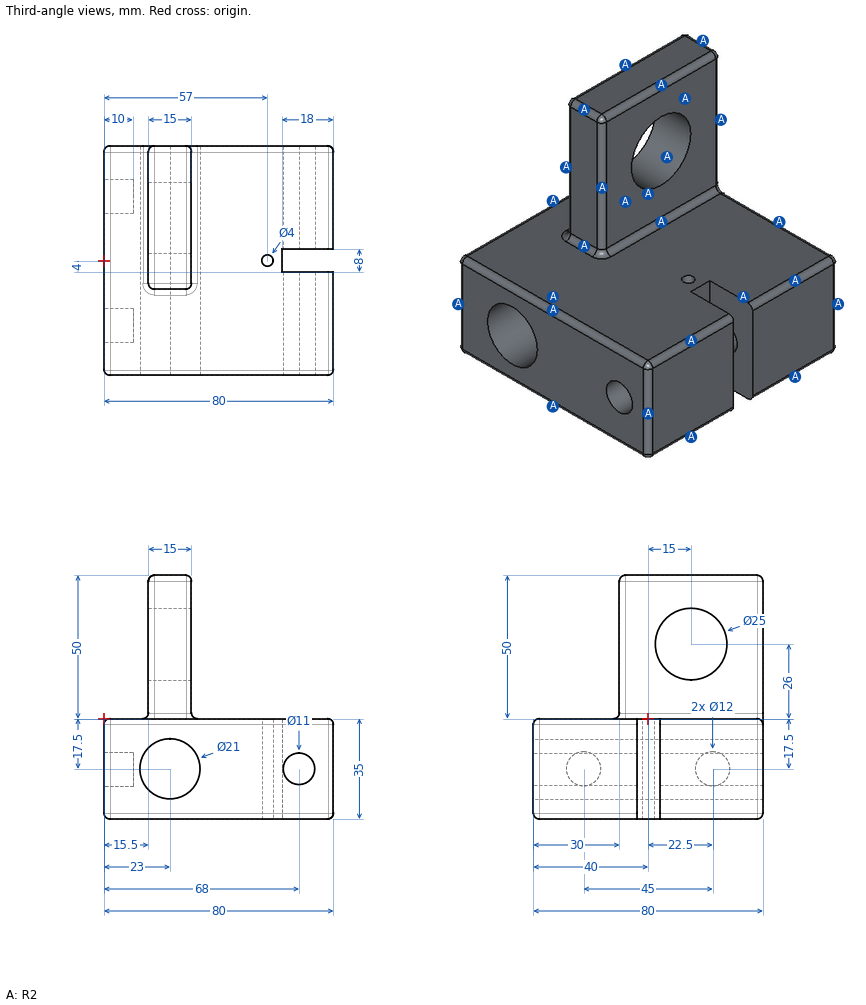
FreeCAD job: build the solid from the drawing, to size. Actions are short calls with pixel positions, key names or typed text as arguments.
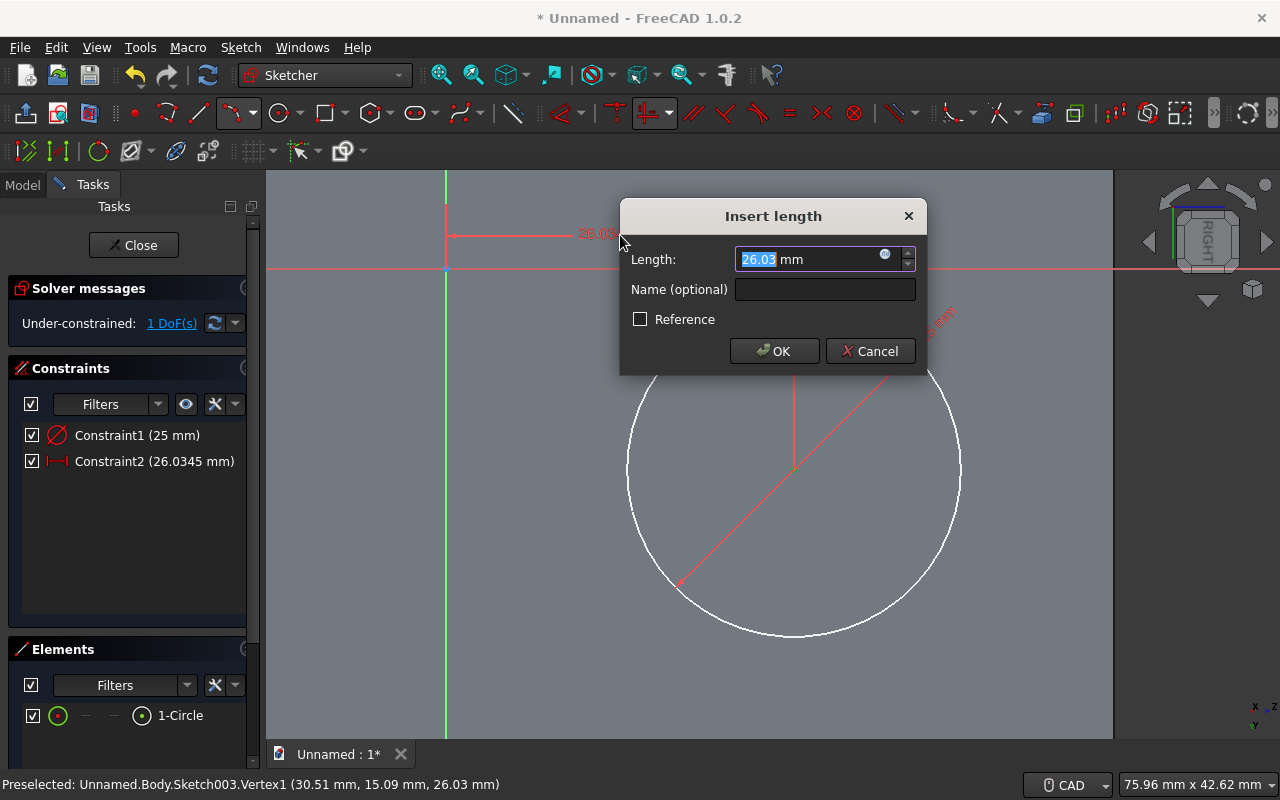
text(26)
key(Return)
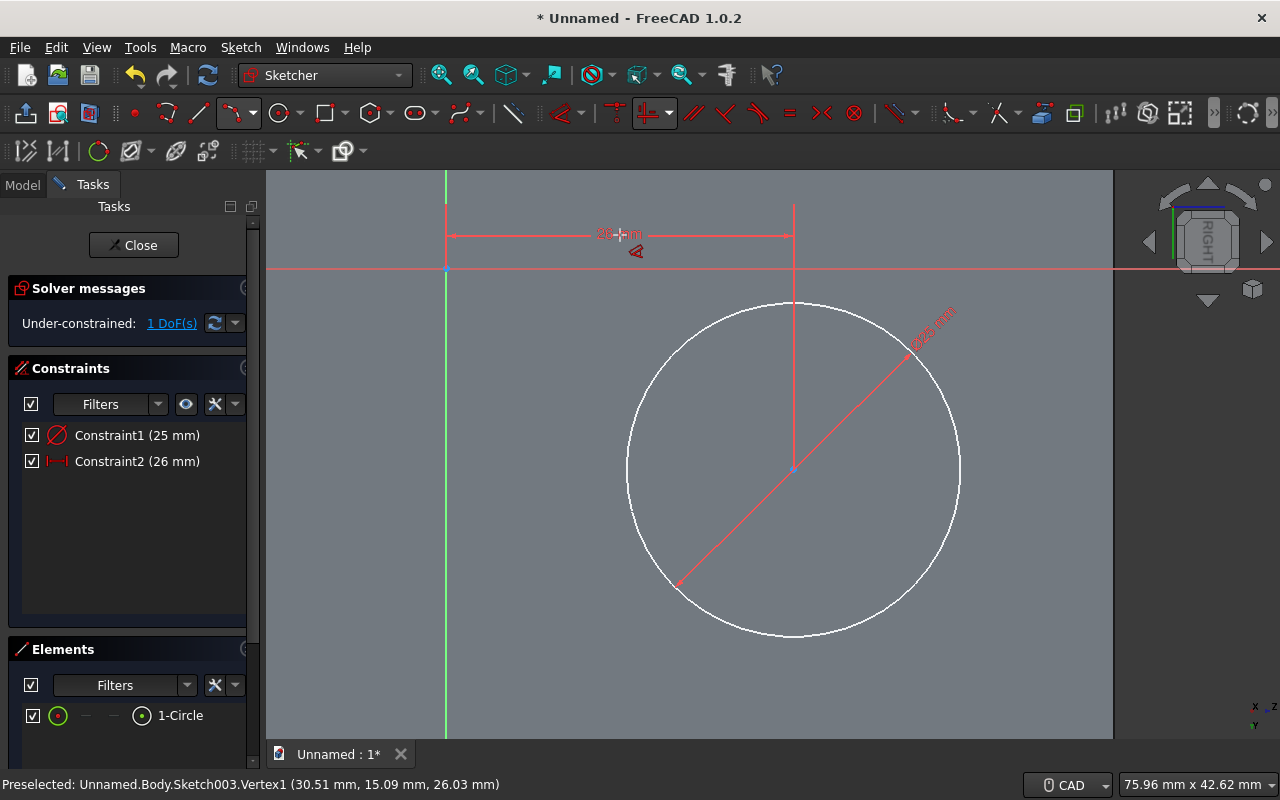
click(794, 470)
click(412, 369)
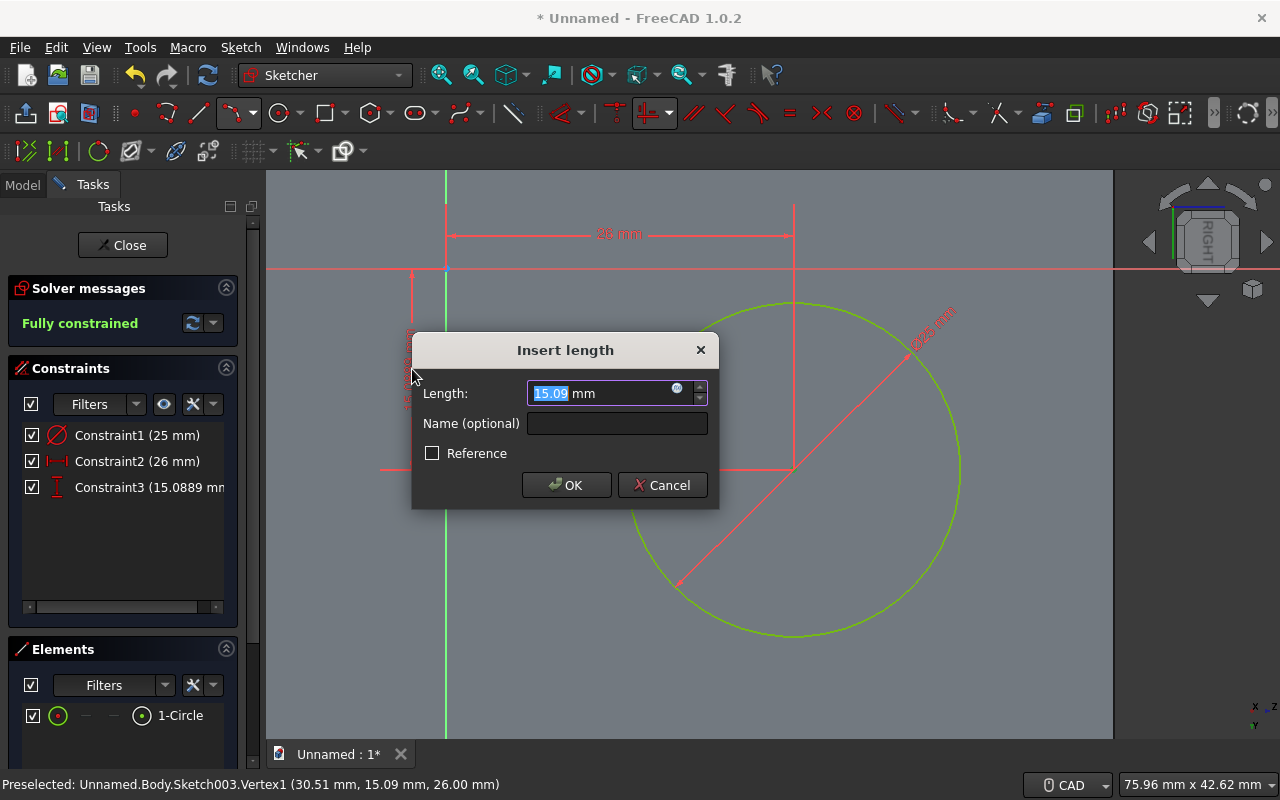
text(15)
key(Return)
key(Escape)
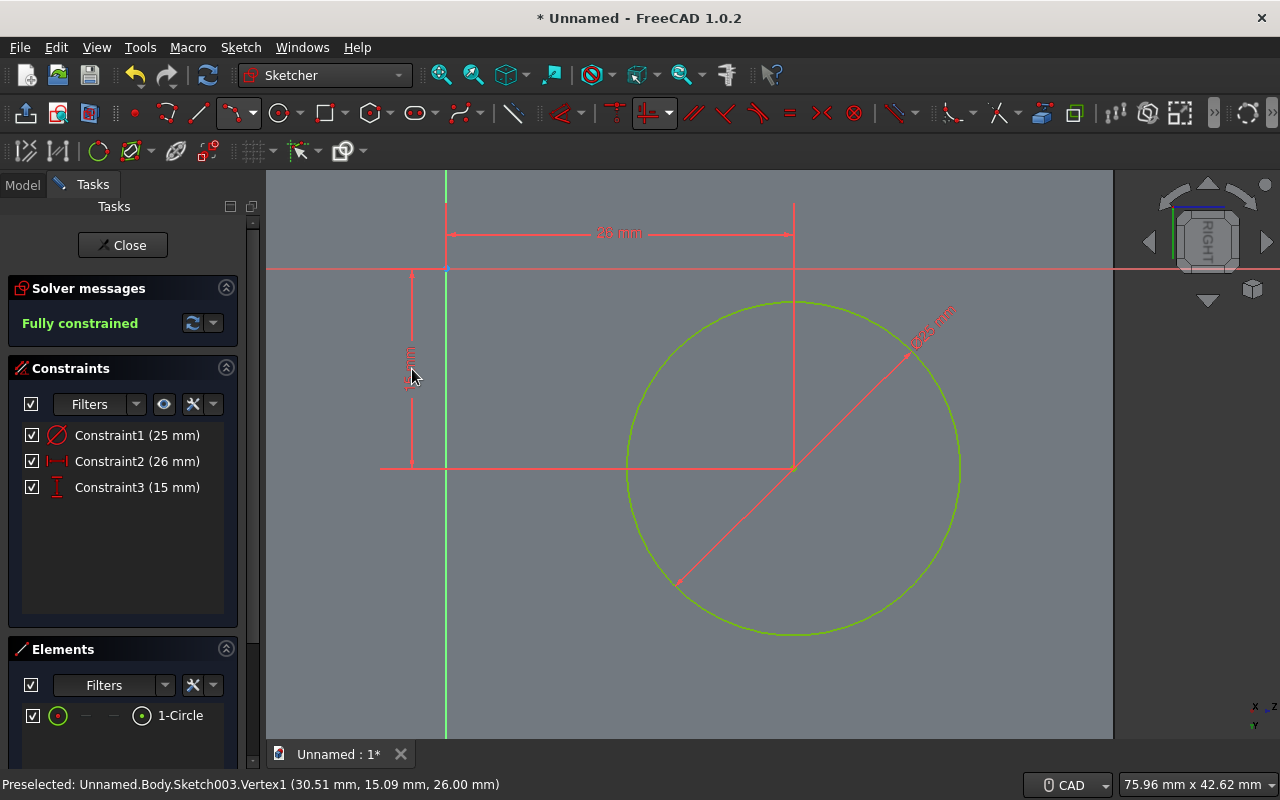
click(123, 245)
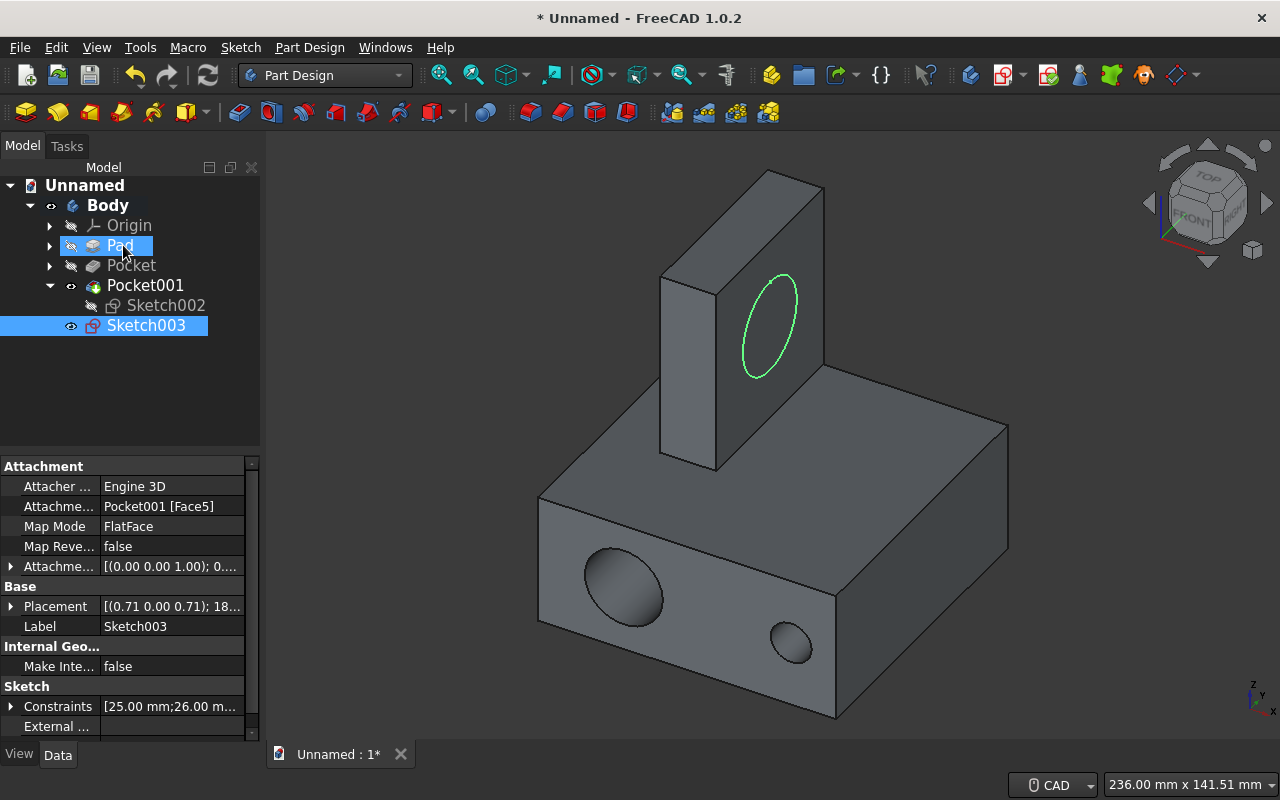
click(240, 112)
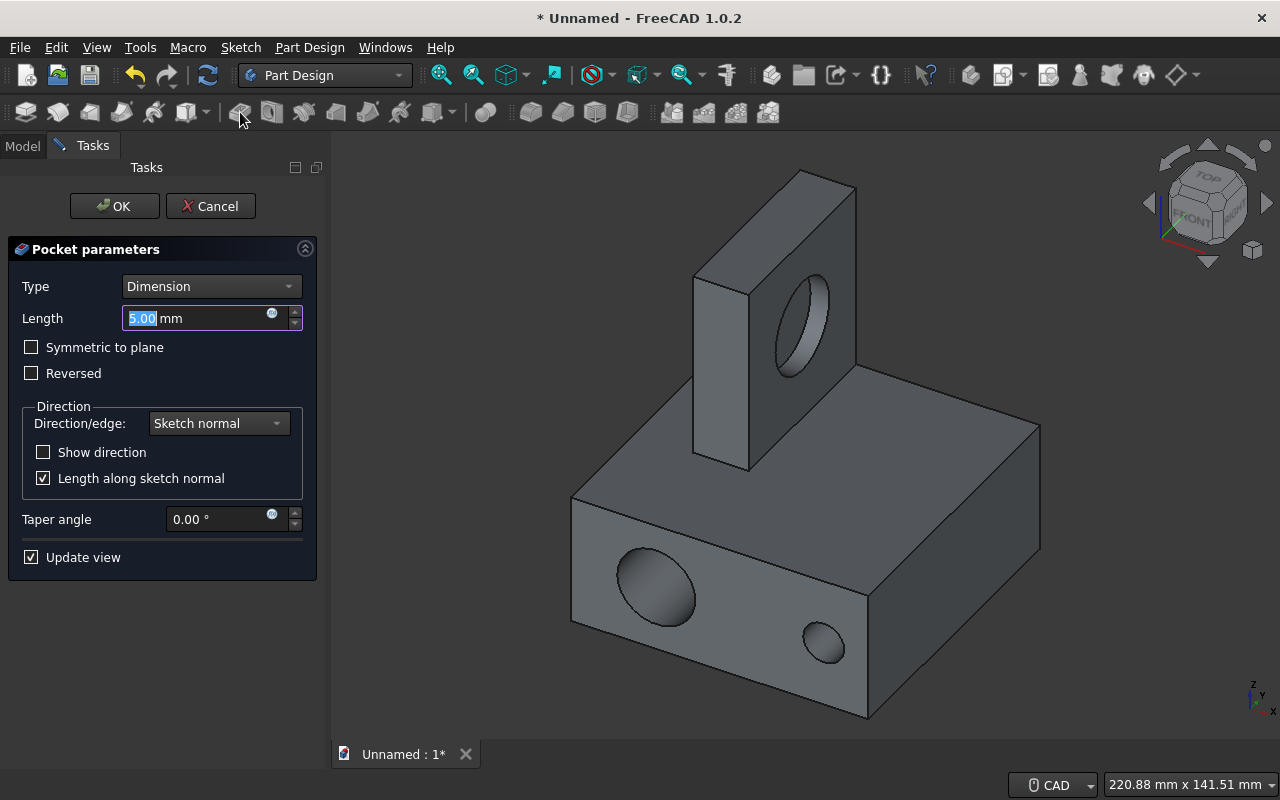
text(15)
key(Tab)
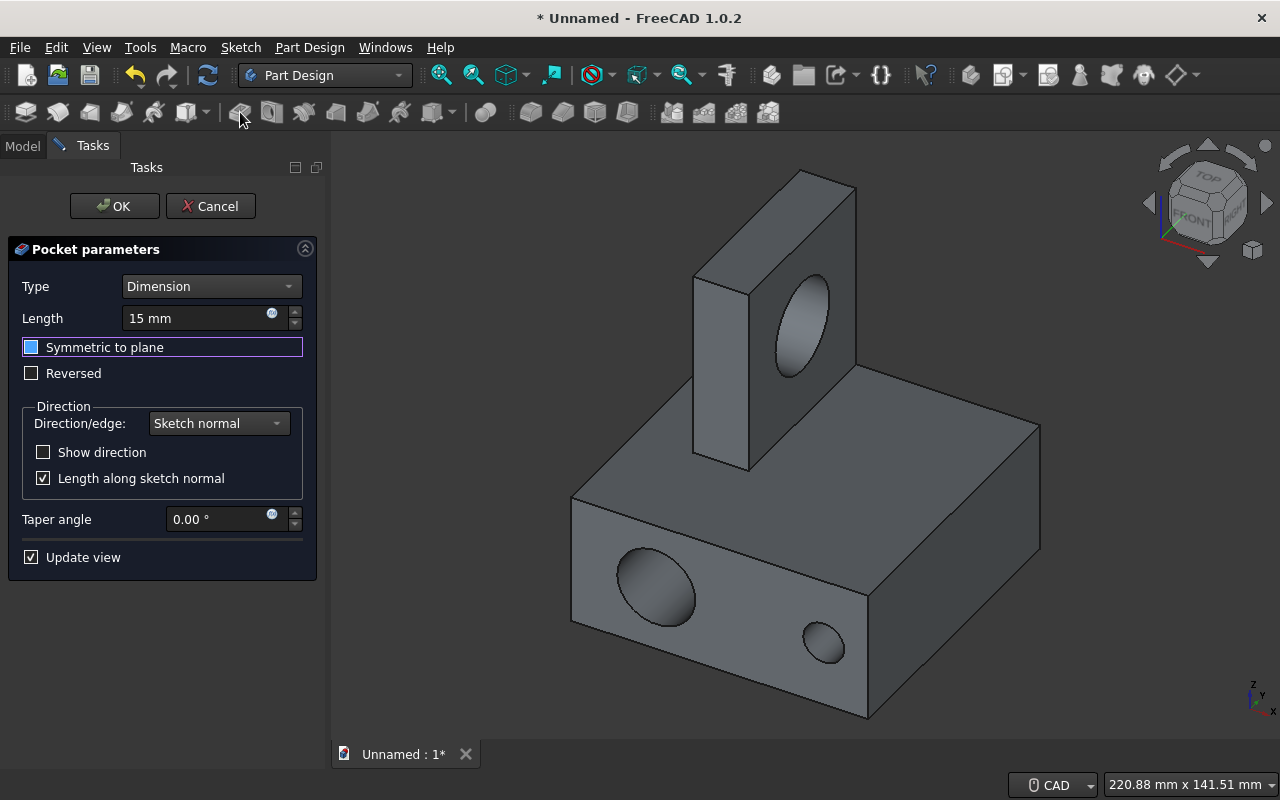
click(115, 206)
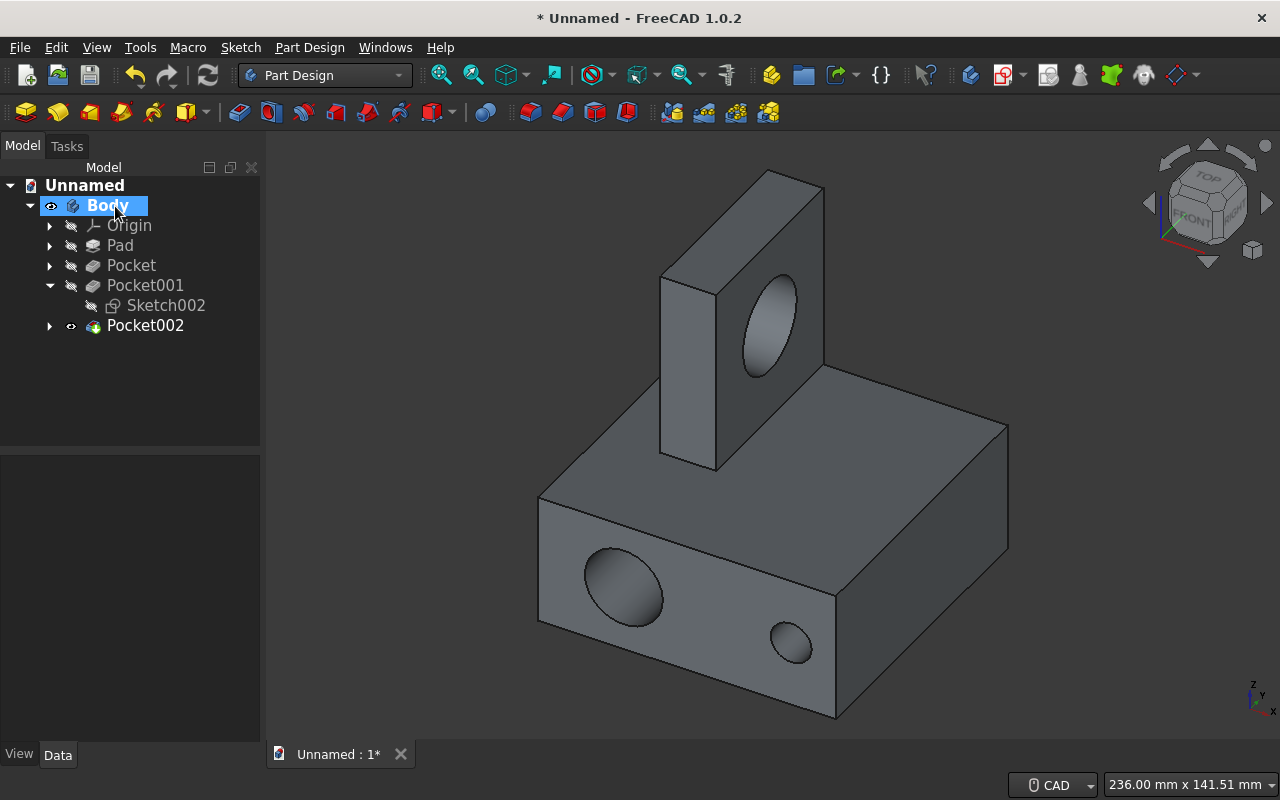
click(791, 499)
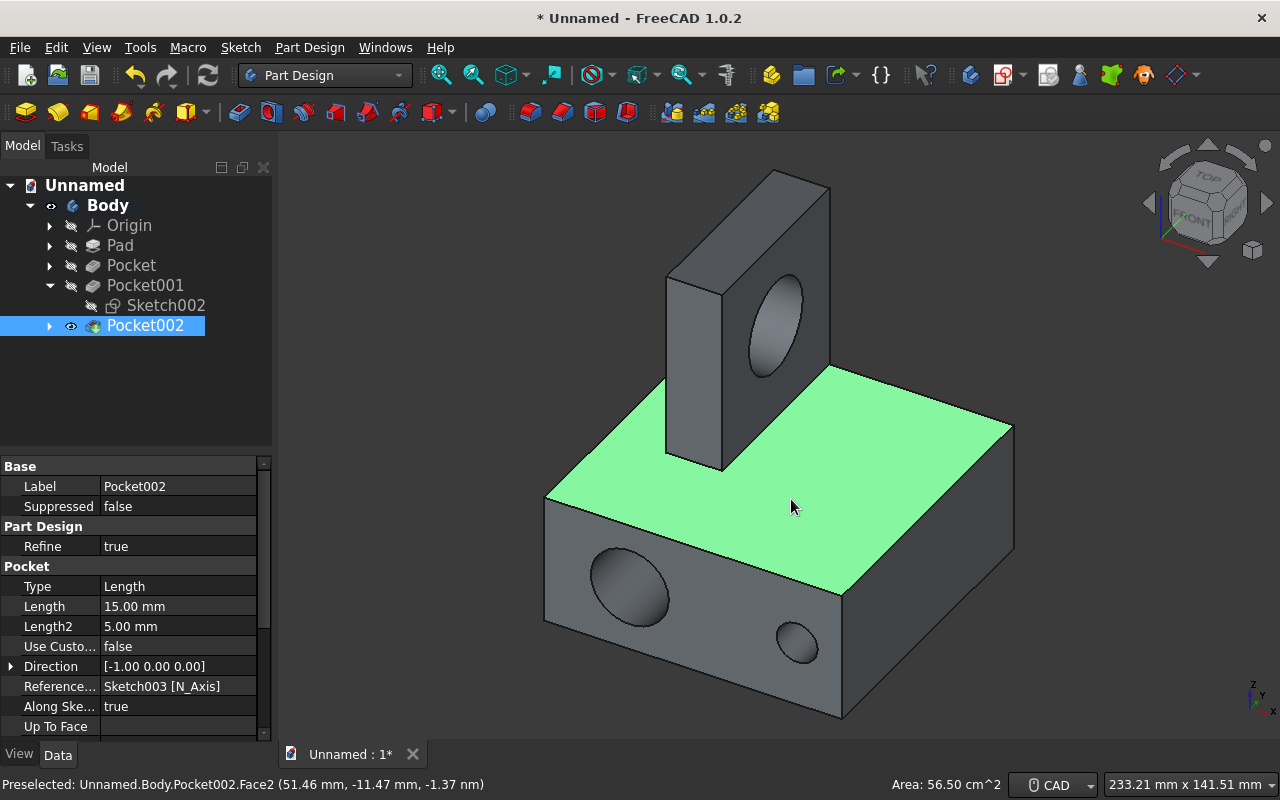
click(1004, 76)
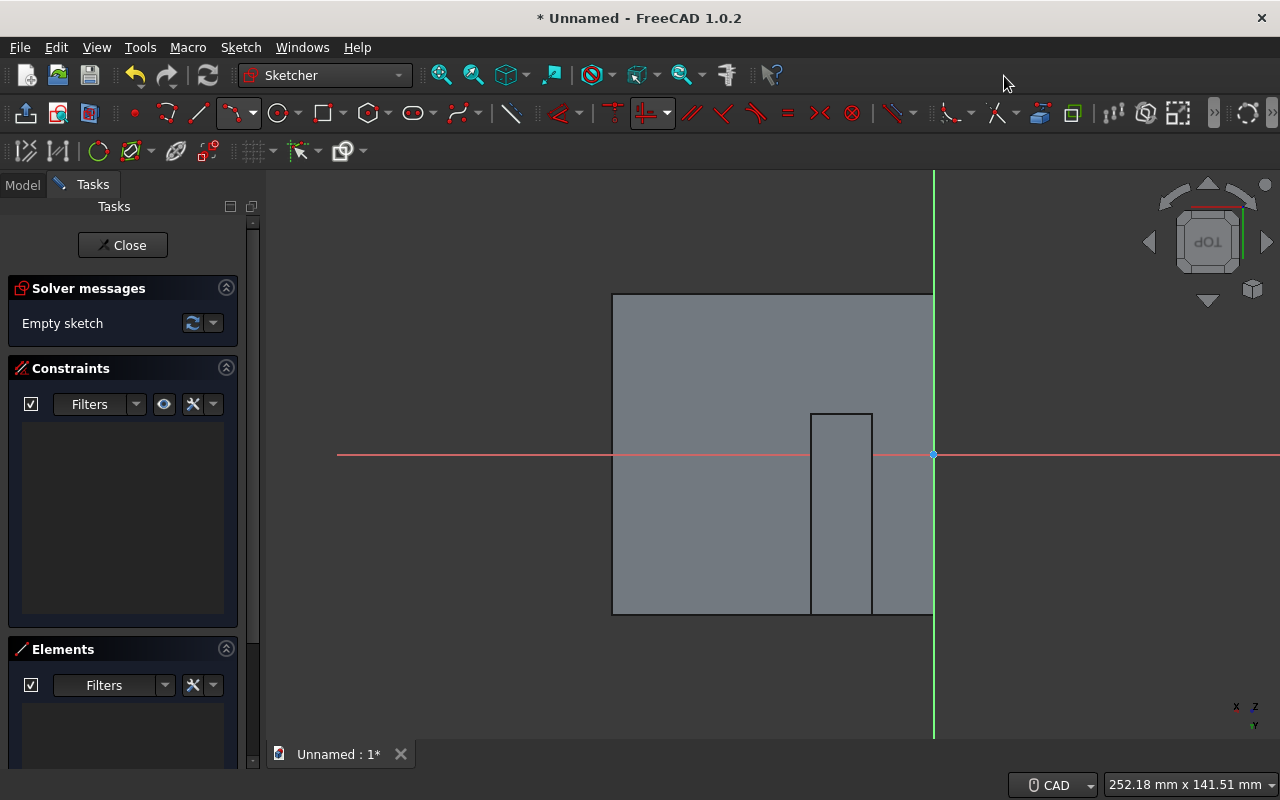
scroll(640, 455, up, 10)